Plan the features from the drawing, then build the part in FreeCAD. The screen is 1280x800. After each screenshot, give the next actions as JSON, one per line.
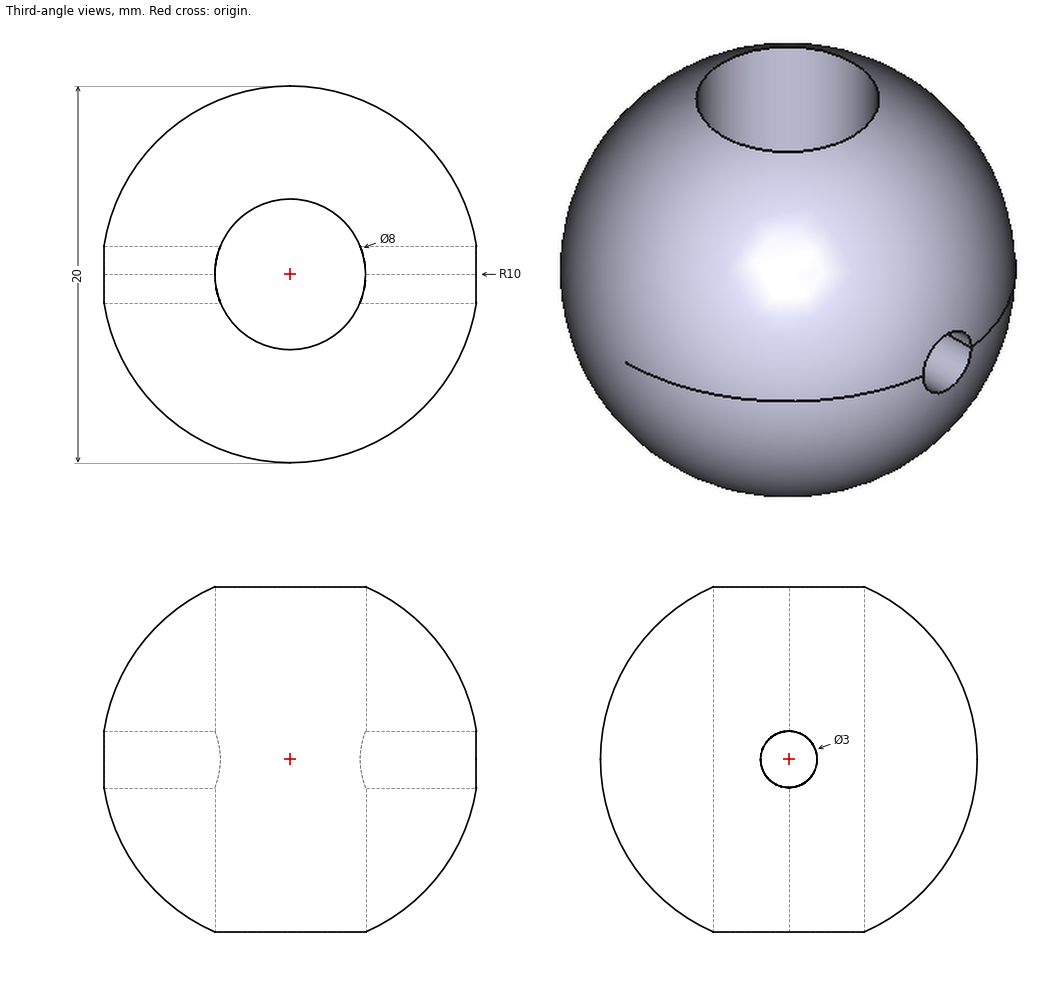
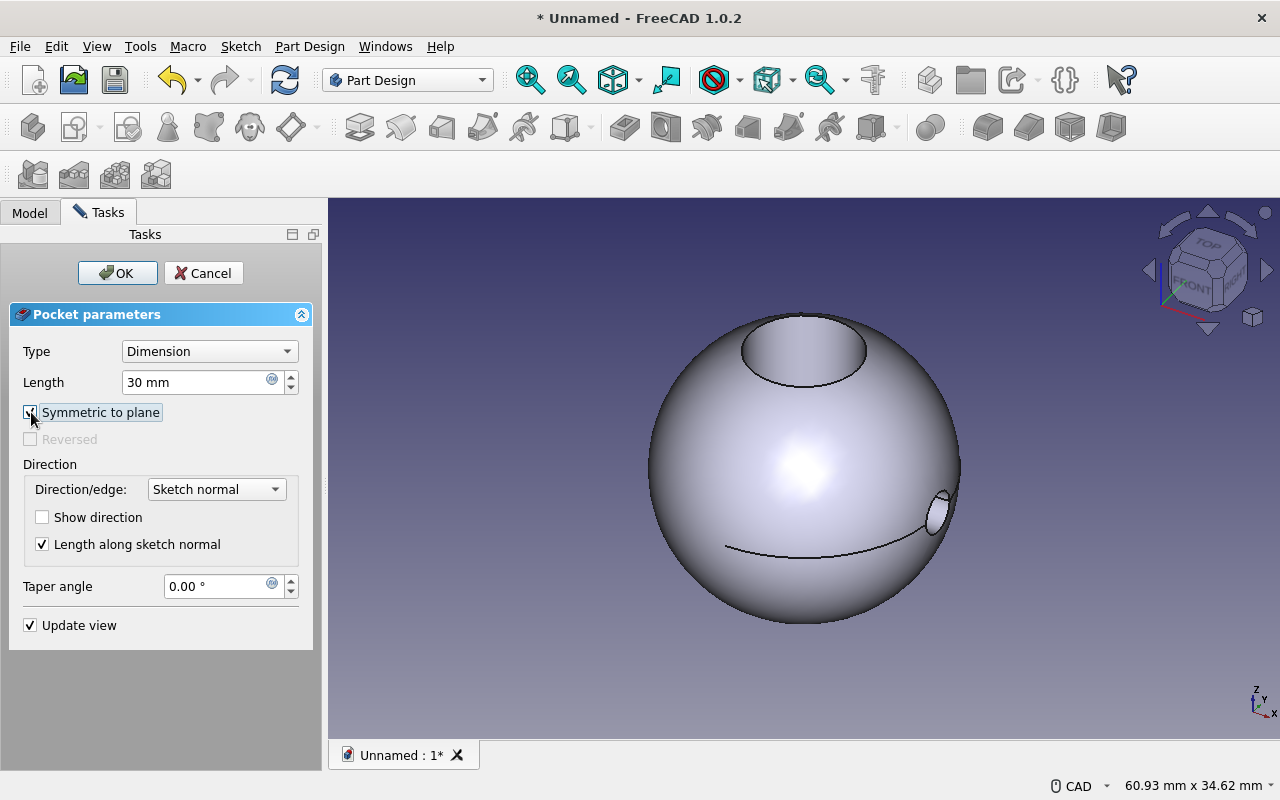
{"action": "left_click", "coordinate": [118, 273]}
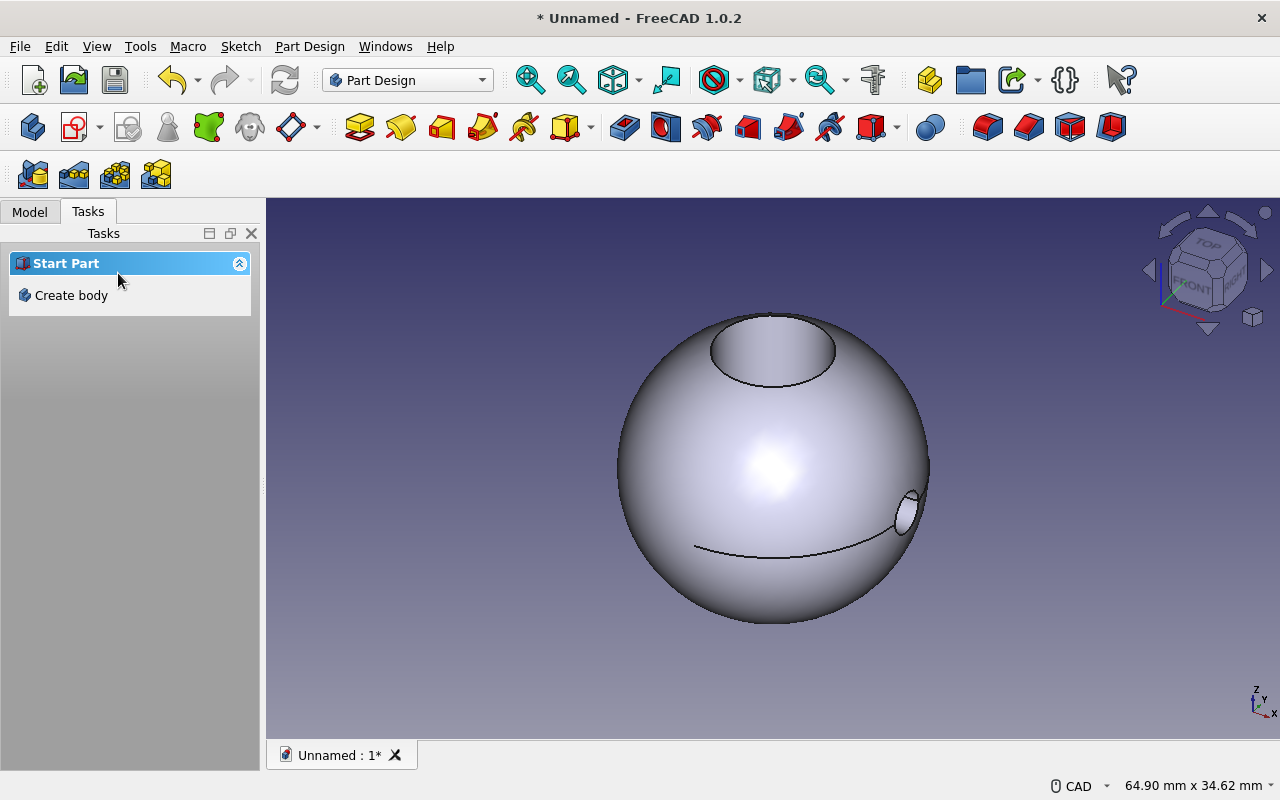
{"action": "key", "text": "0"}